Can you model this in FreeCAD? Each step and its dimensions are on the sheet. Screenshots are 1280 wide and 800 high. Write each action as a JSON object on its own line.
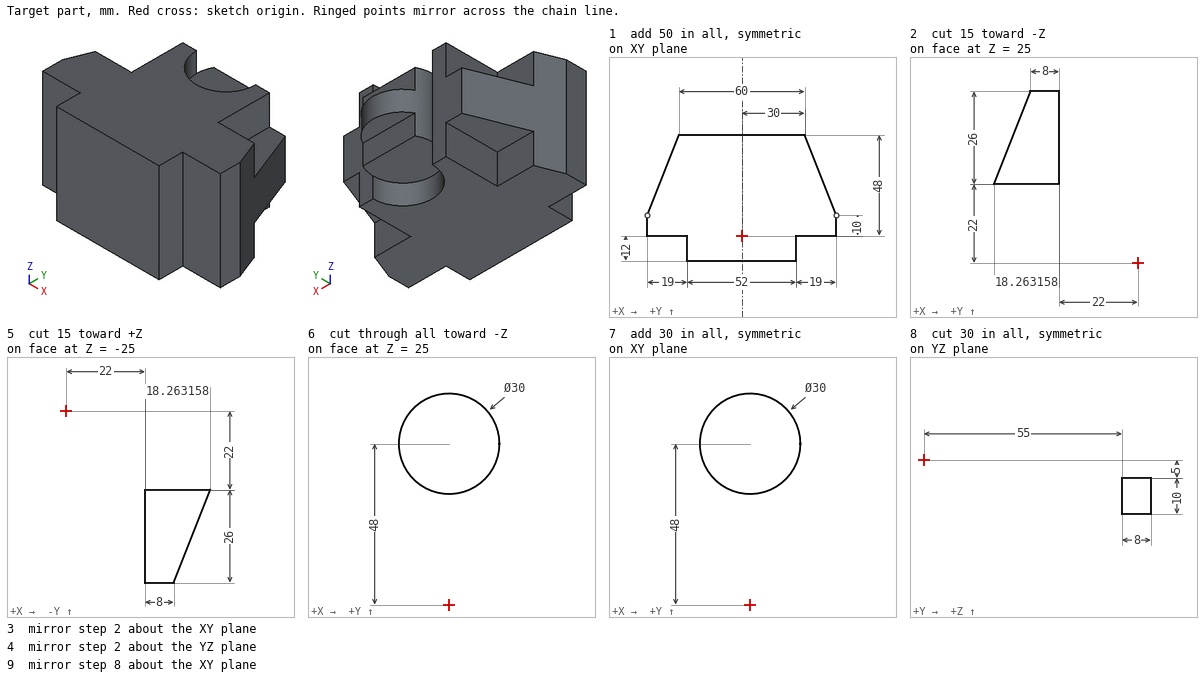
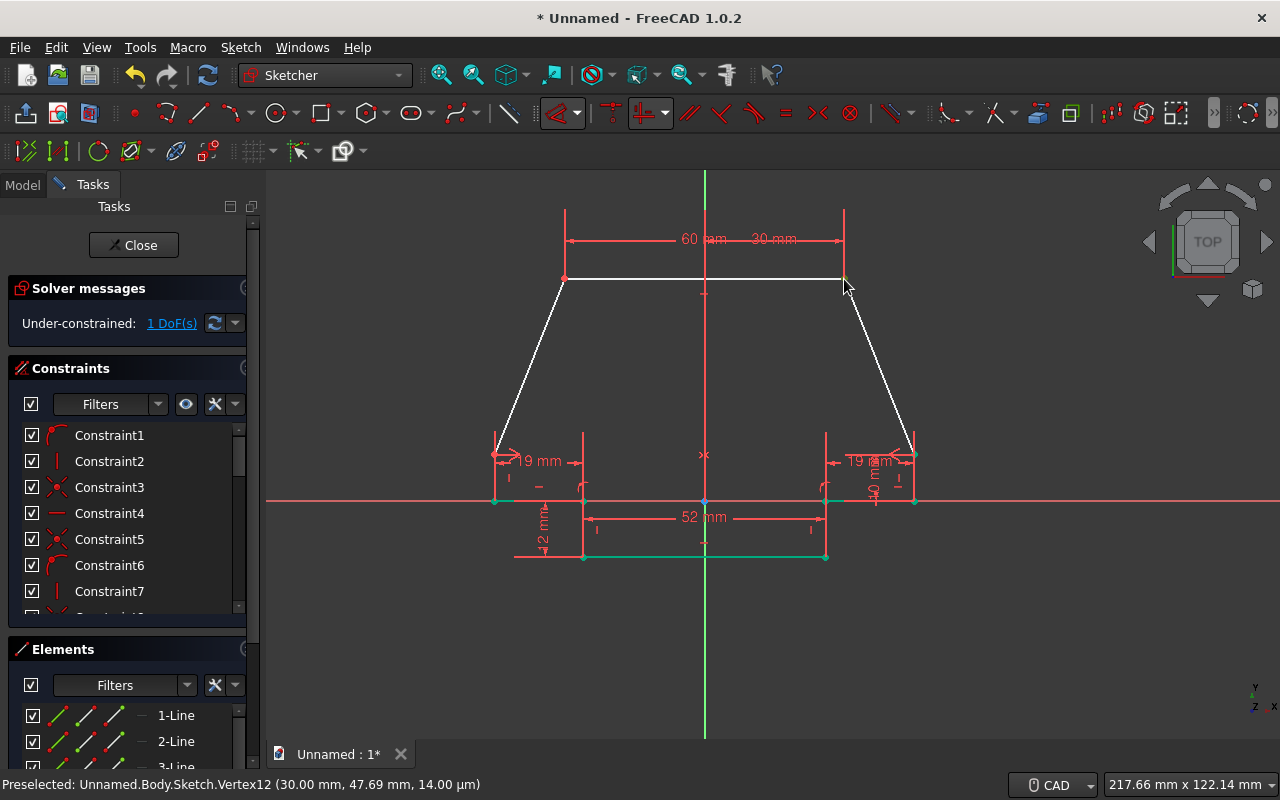
{"action": "left_click", "coordinate": [580, 114]}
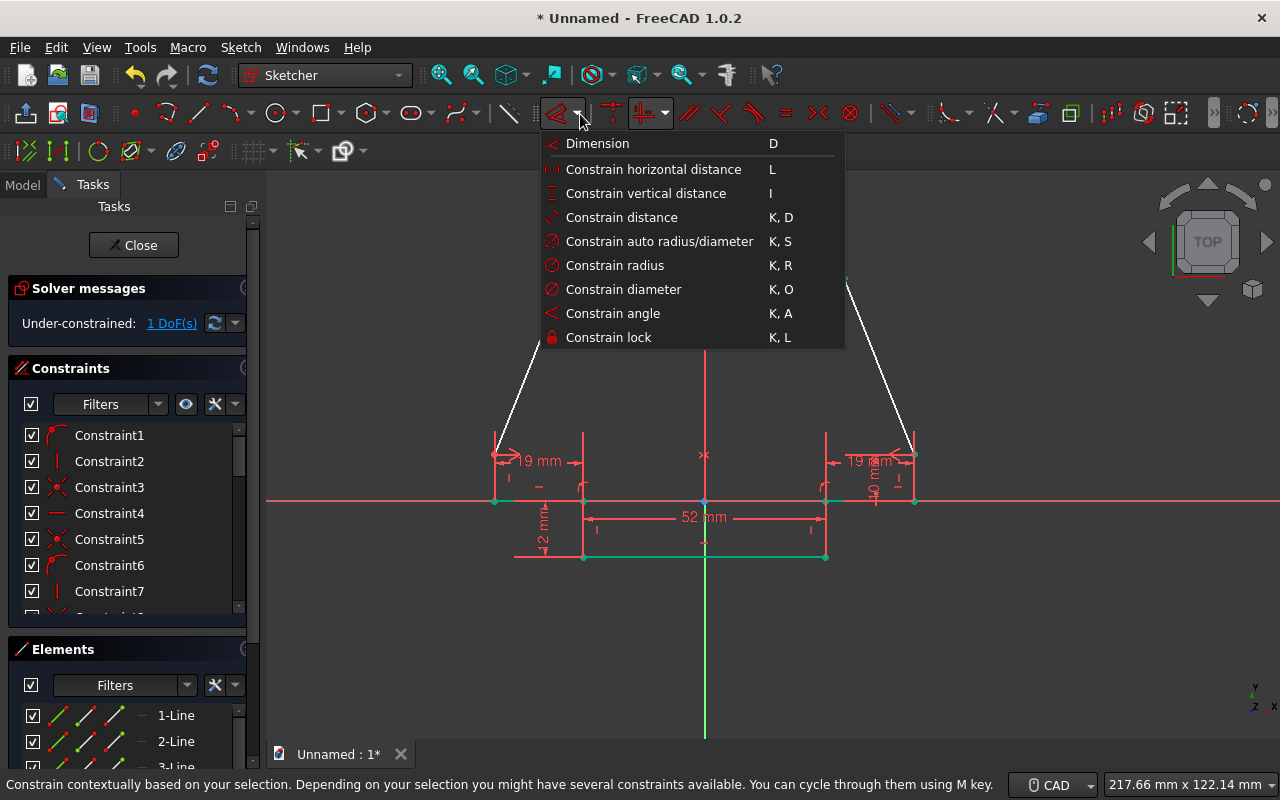
{"action": "left_click", "coordinate": [693, 193]}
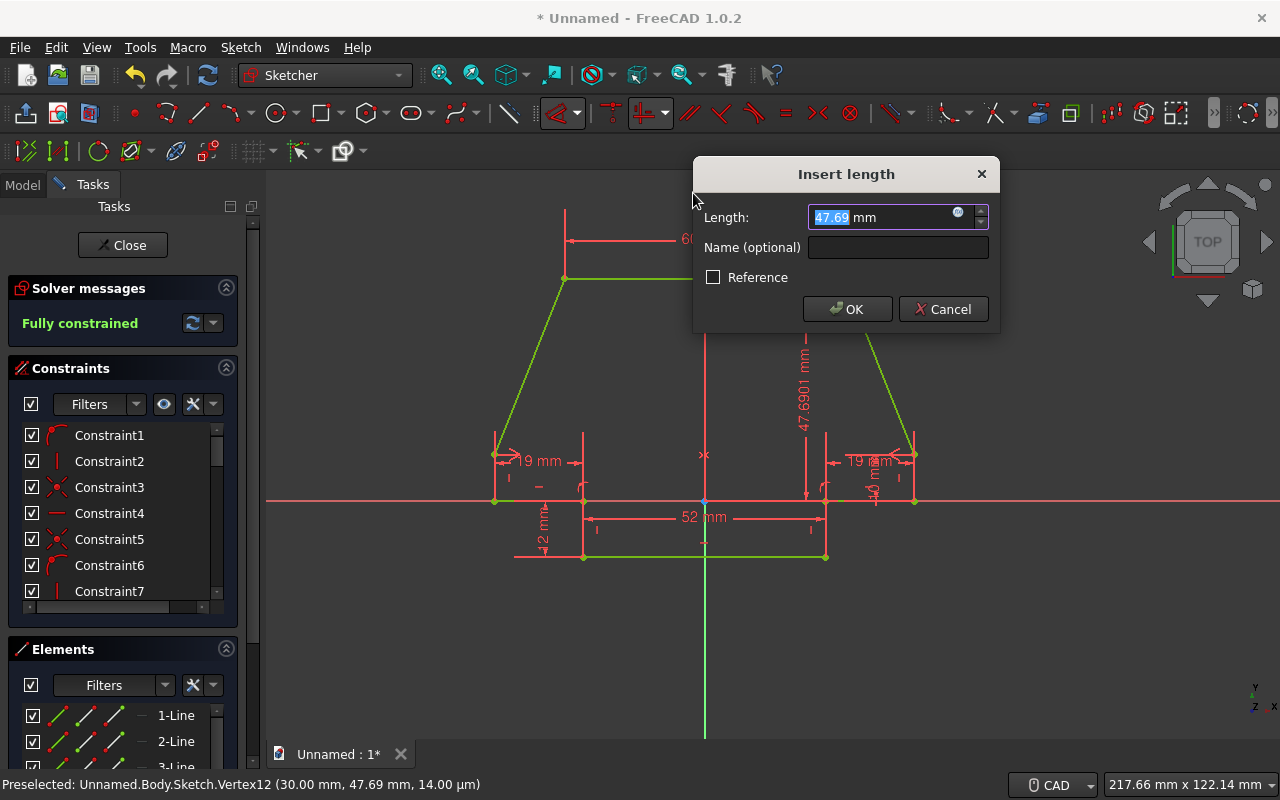
{"action": "type", "text": "48"}
{"action": "key", "text": "Return"}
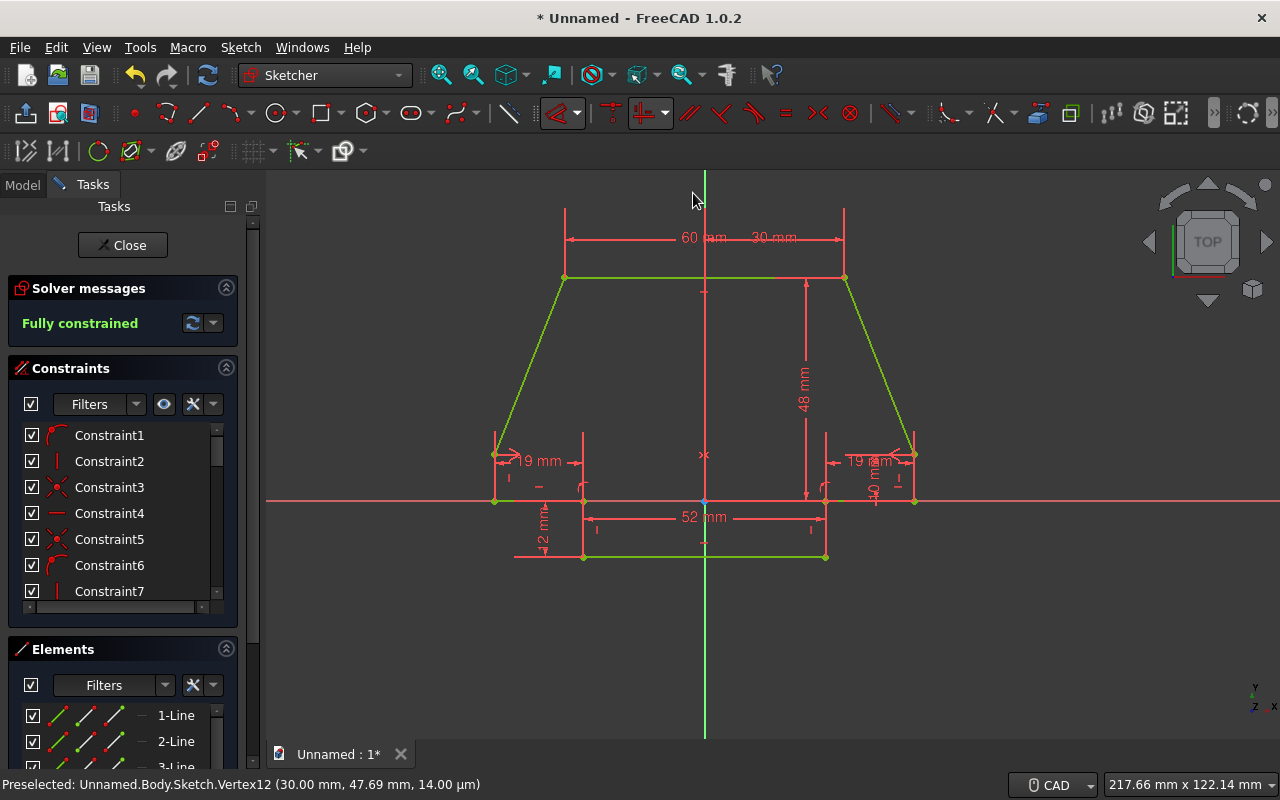
{"action": "left_click", "coordinate": [123, 245]}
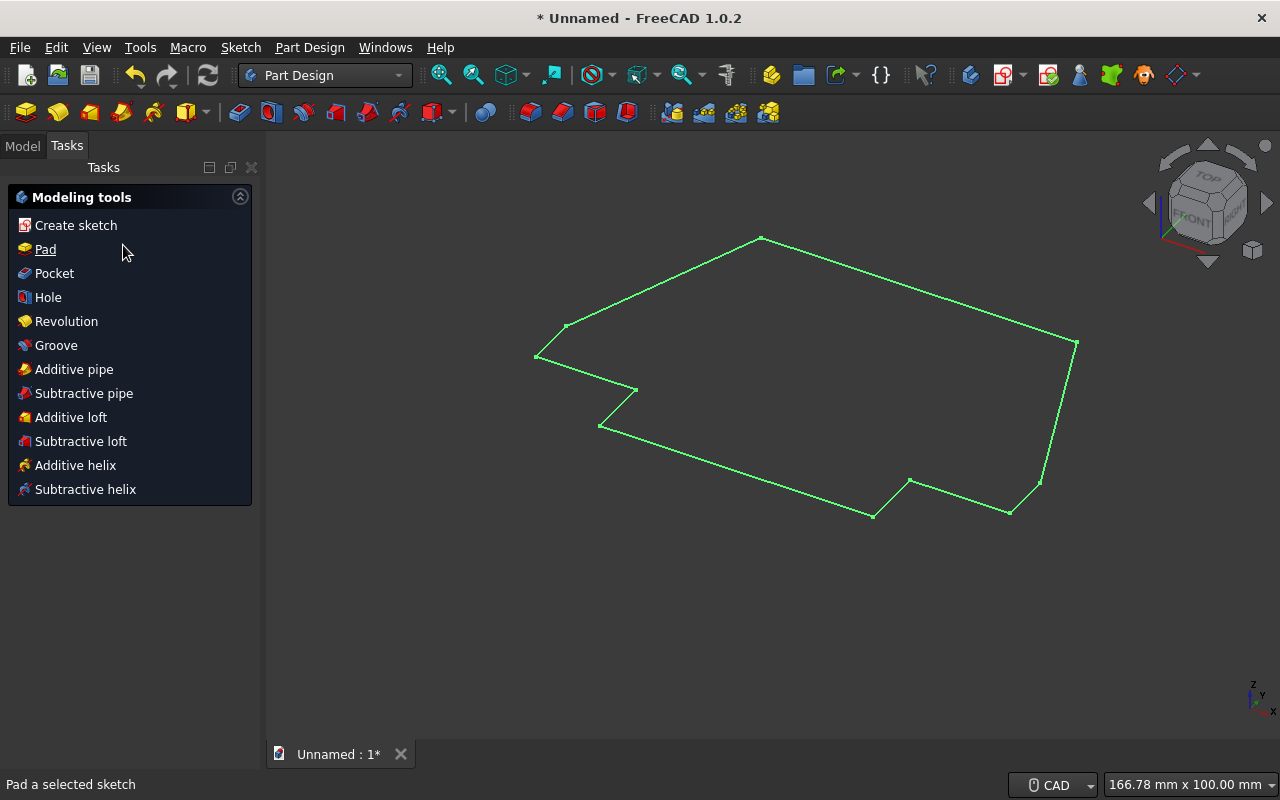
{"action": "left_click", "coordinate": [26, 112]}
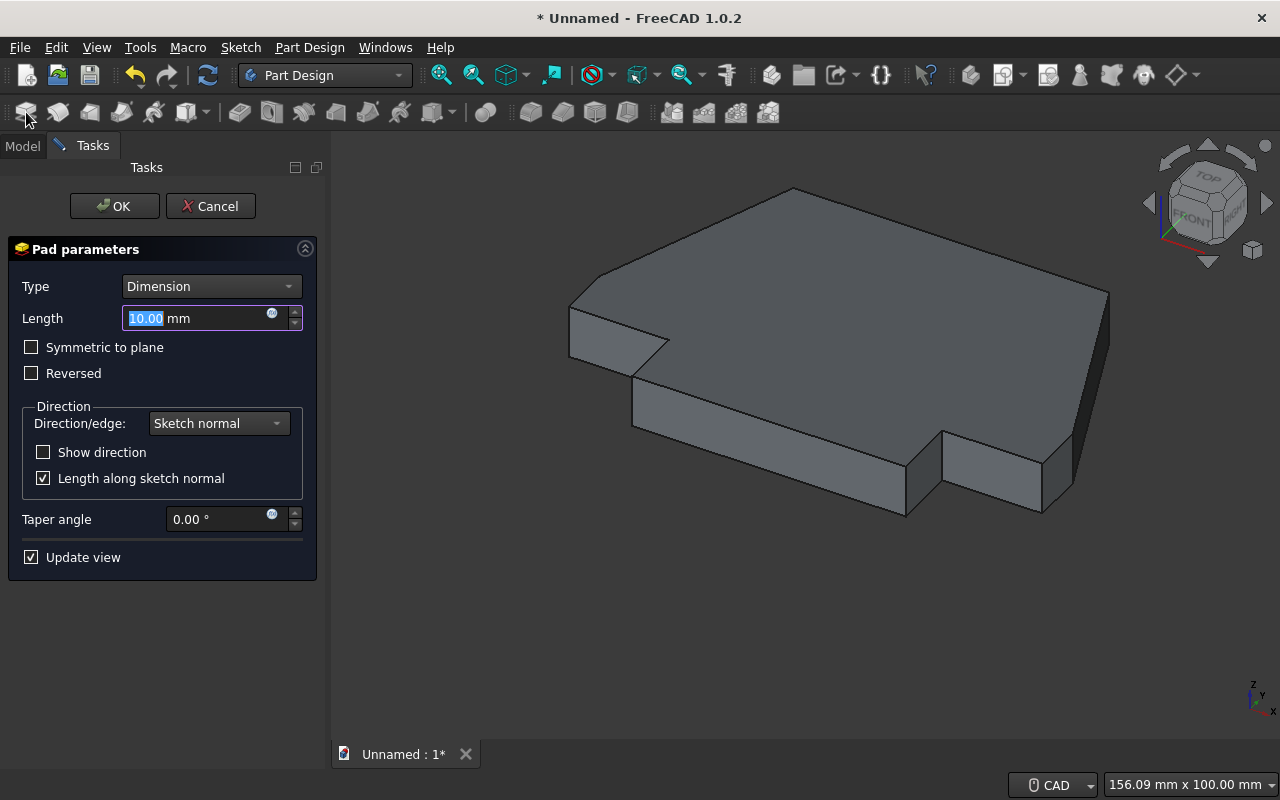
{"action": "type", "text": "50"}
{"action": "key", "text": "Tab"}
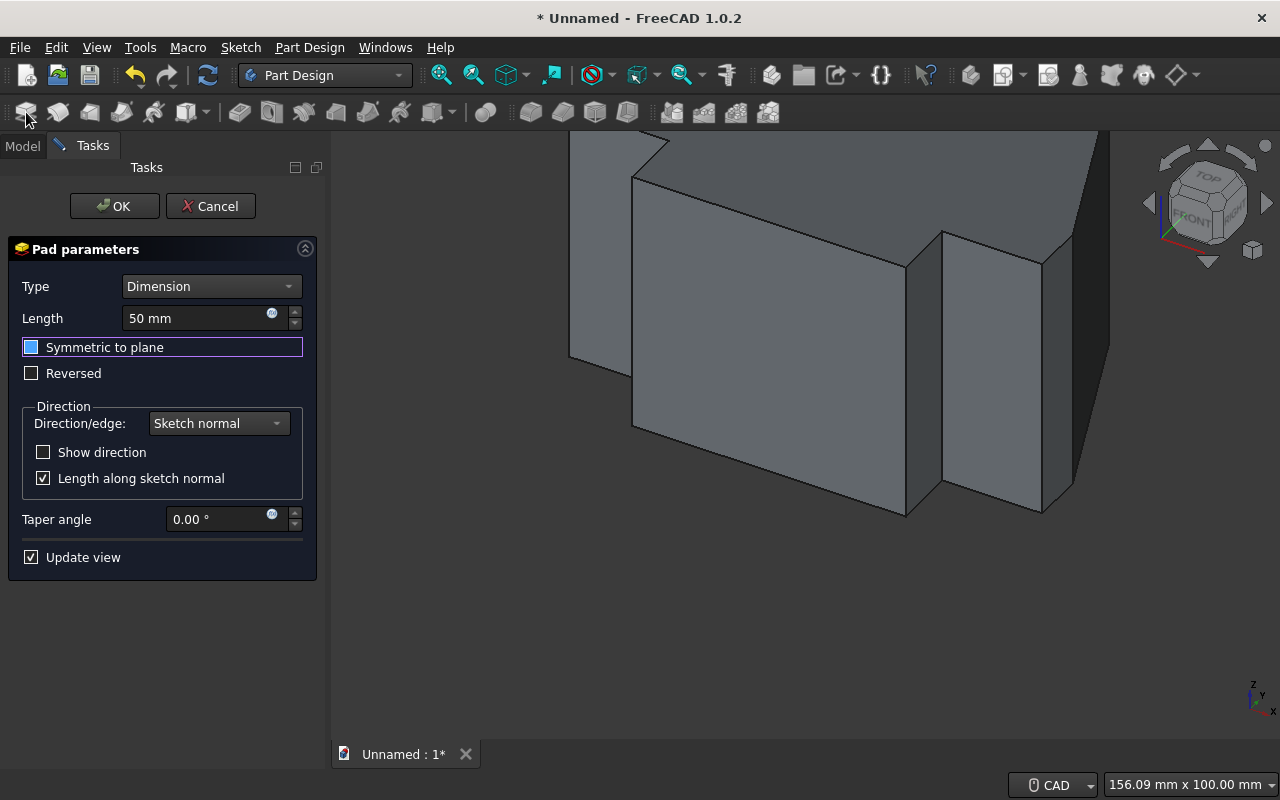
{"action": "left_click", "coordinate": [30, 347]}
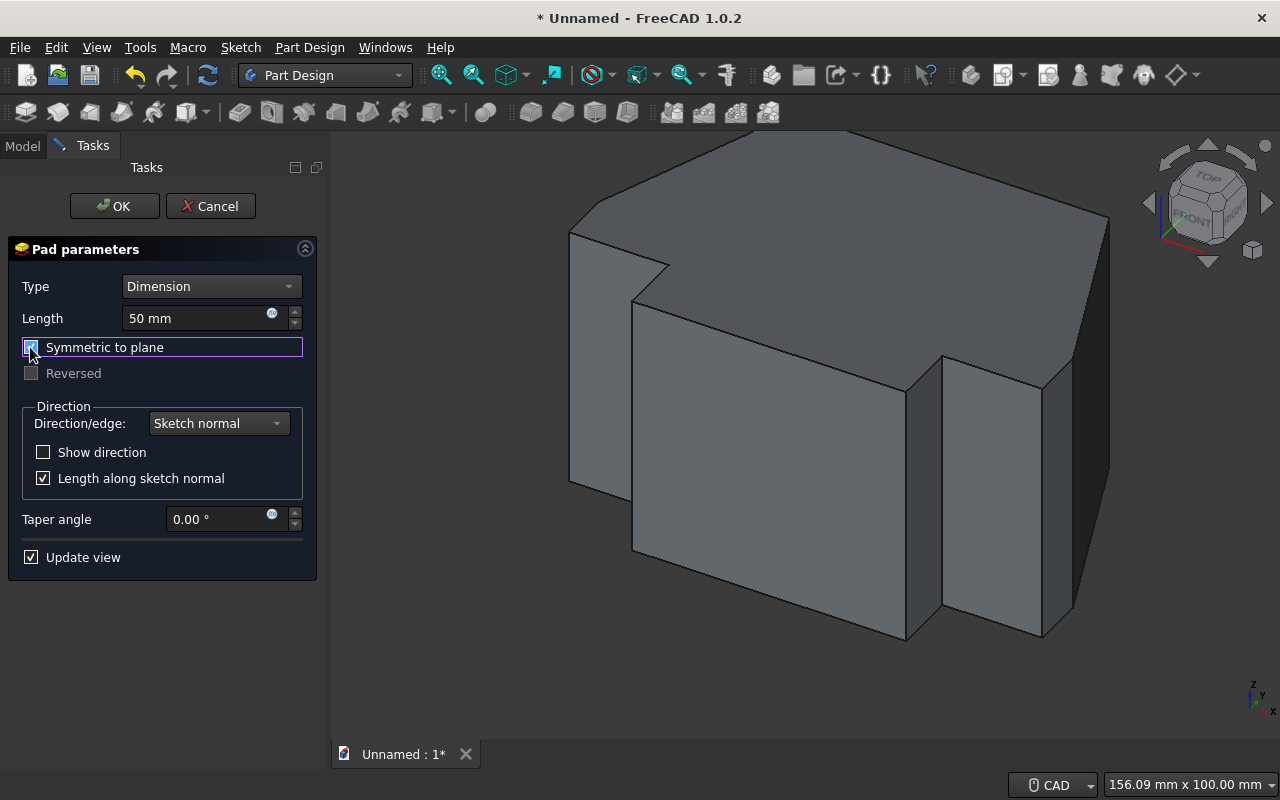
{"action": "left_click", "coordinate": [115, 206]}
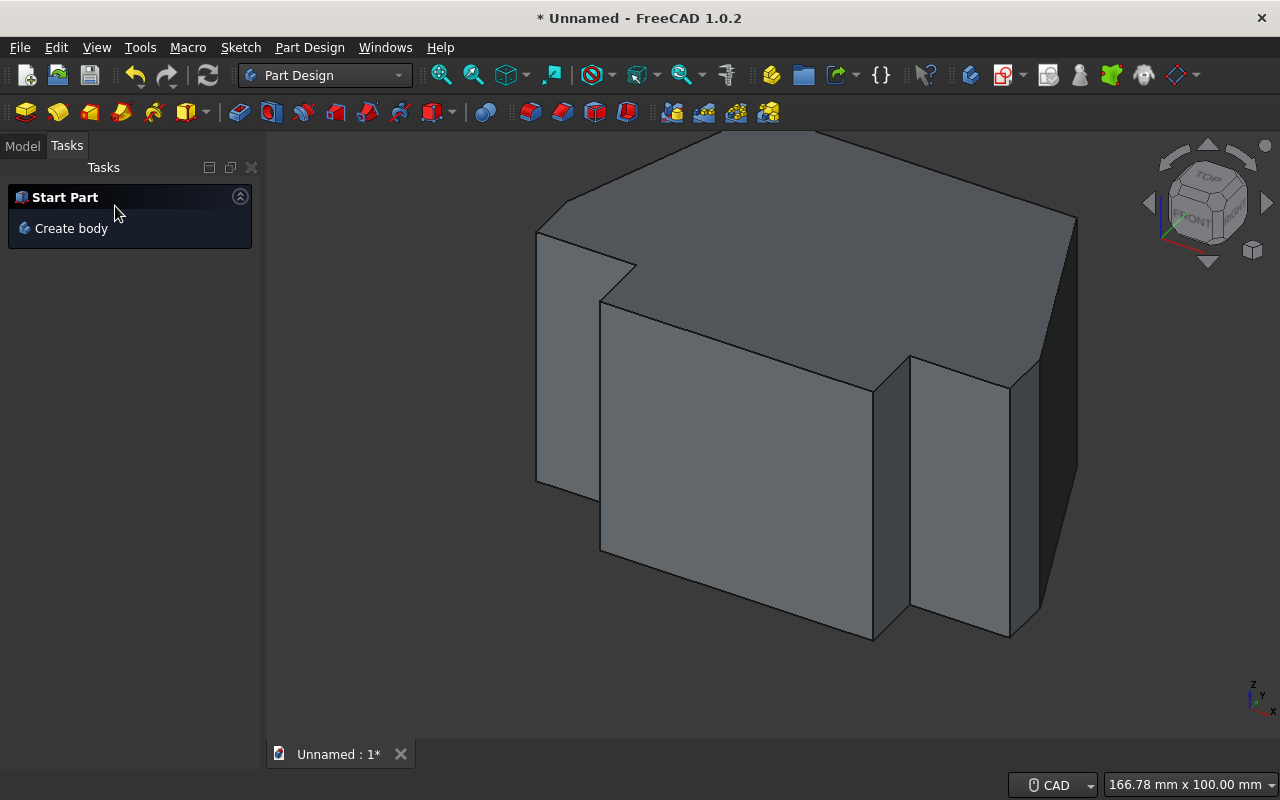
{"action": "left_click", "coordinate": [442, 76]}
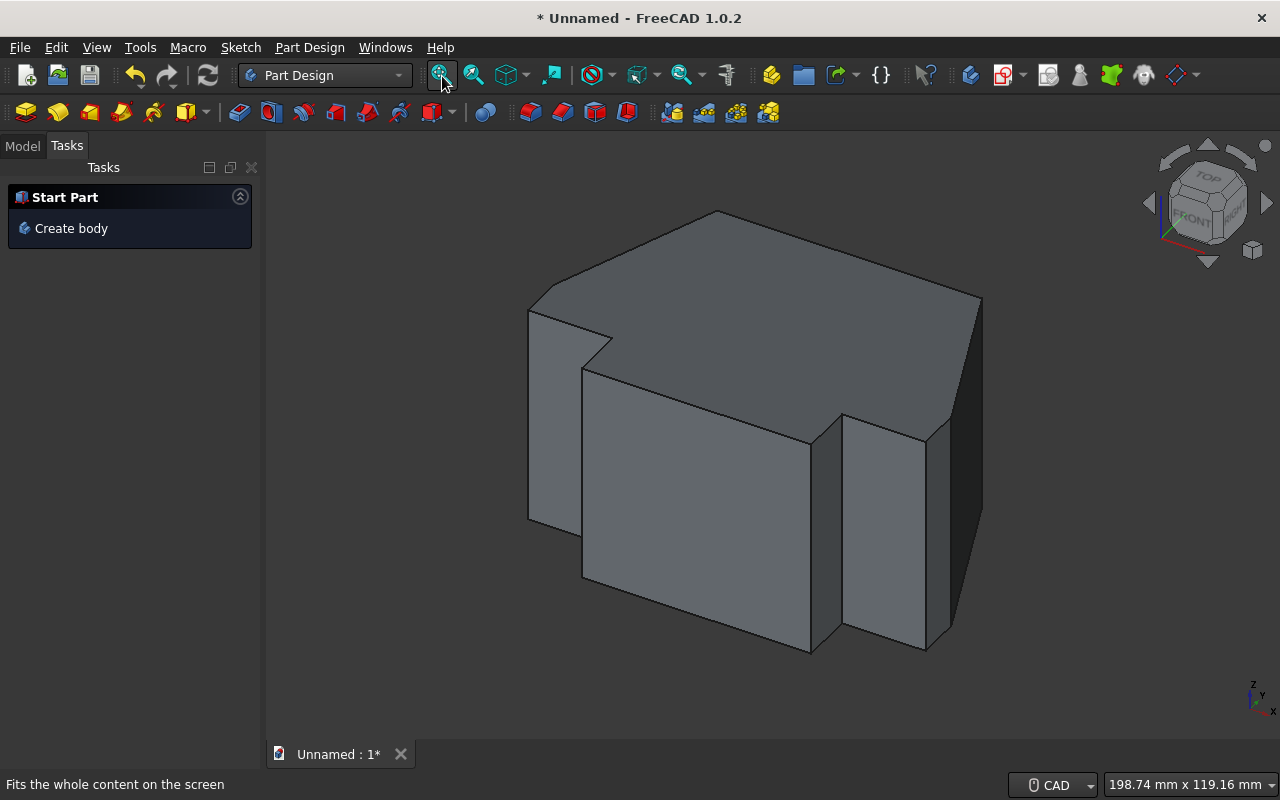
{"action": "left_click", "coordinate": [773, 330]}